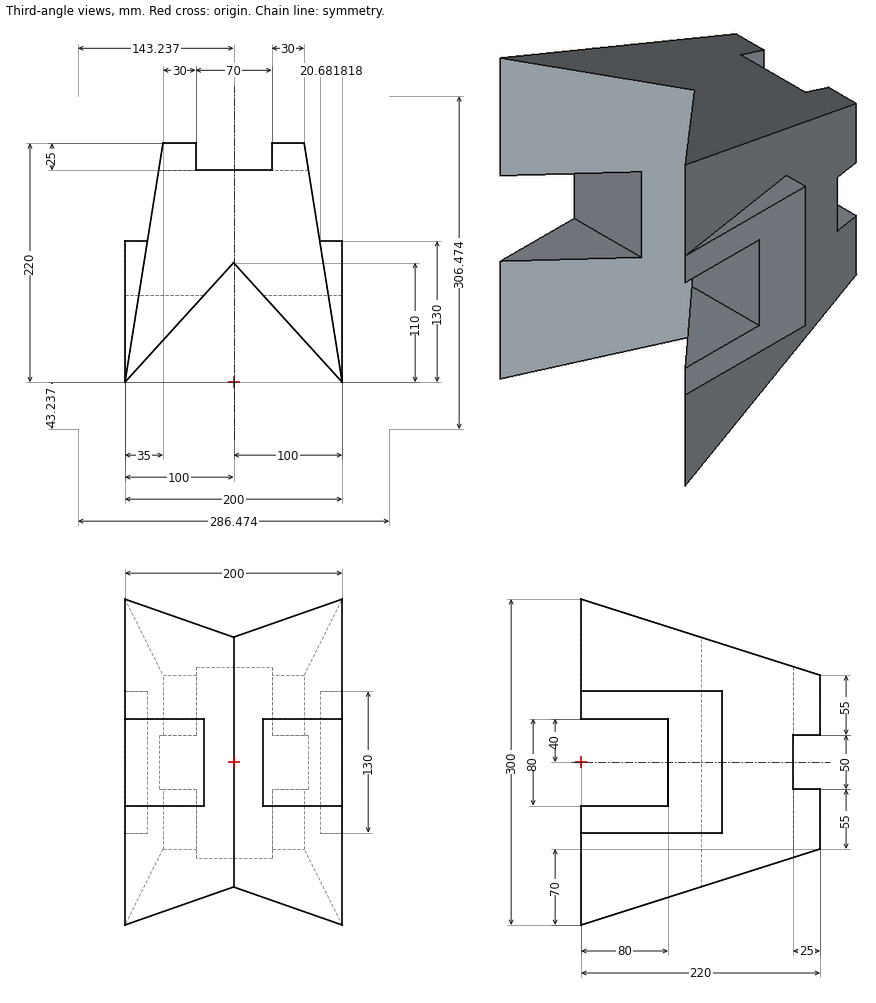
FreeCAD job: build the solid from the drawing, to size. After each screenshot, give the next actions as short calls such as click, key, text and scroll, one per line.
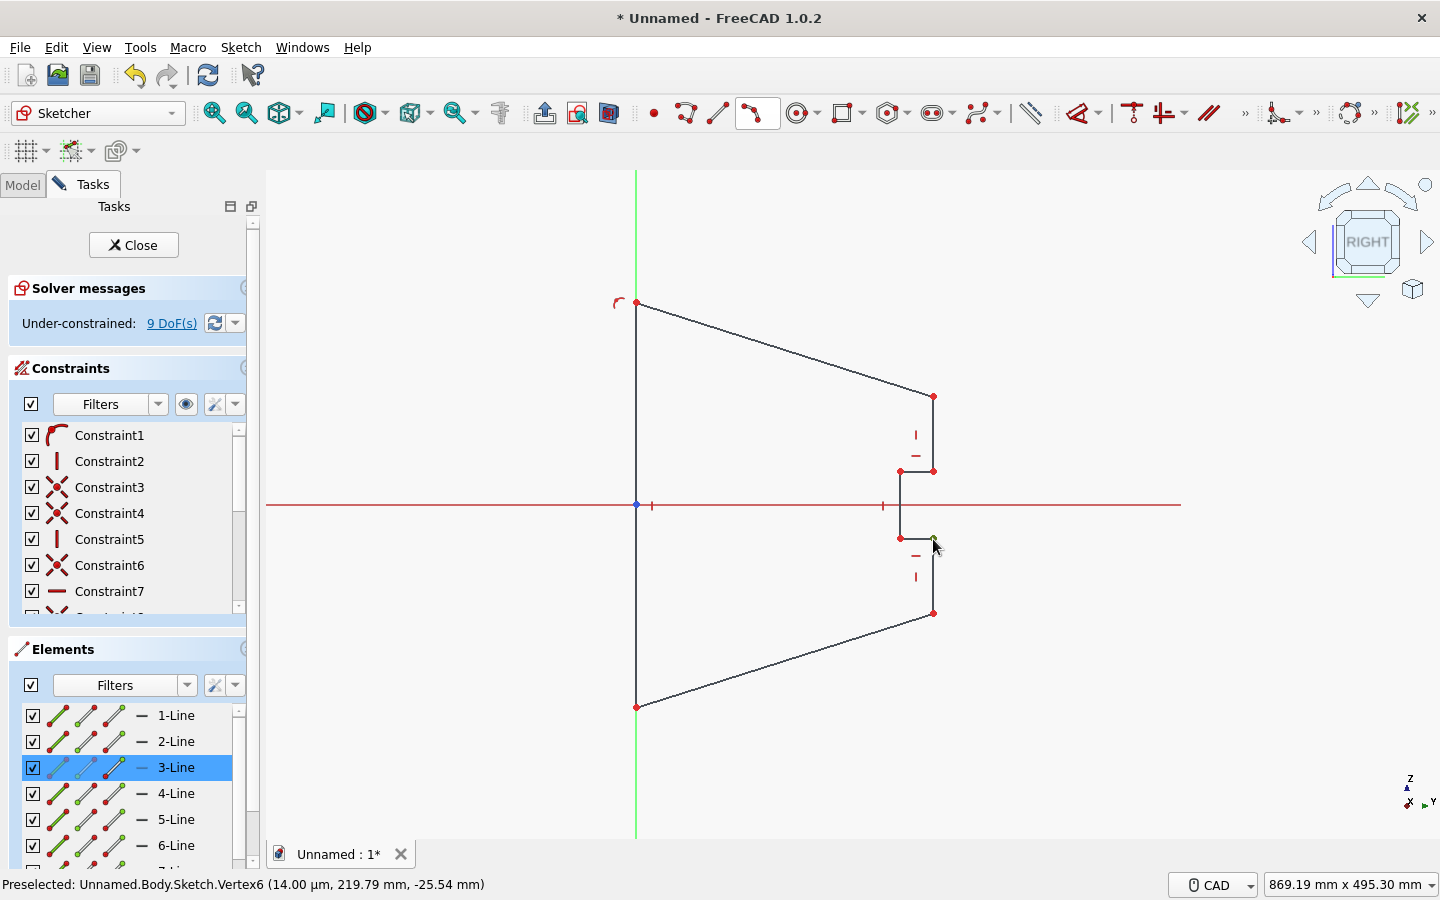
click(933, 472)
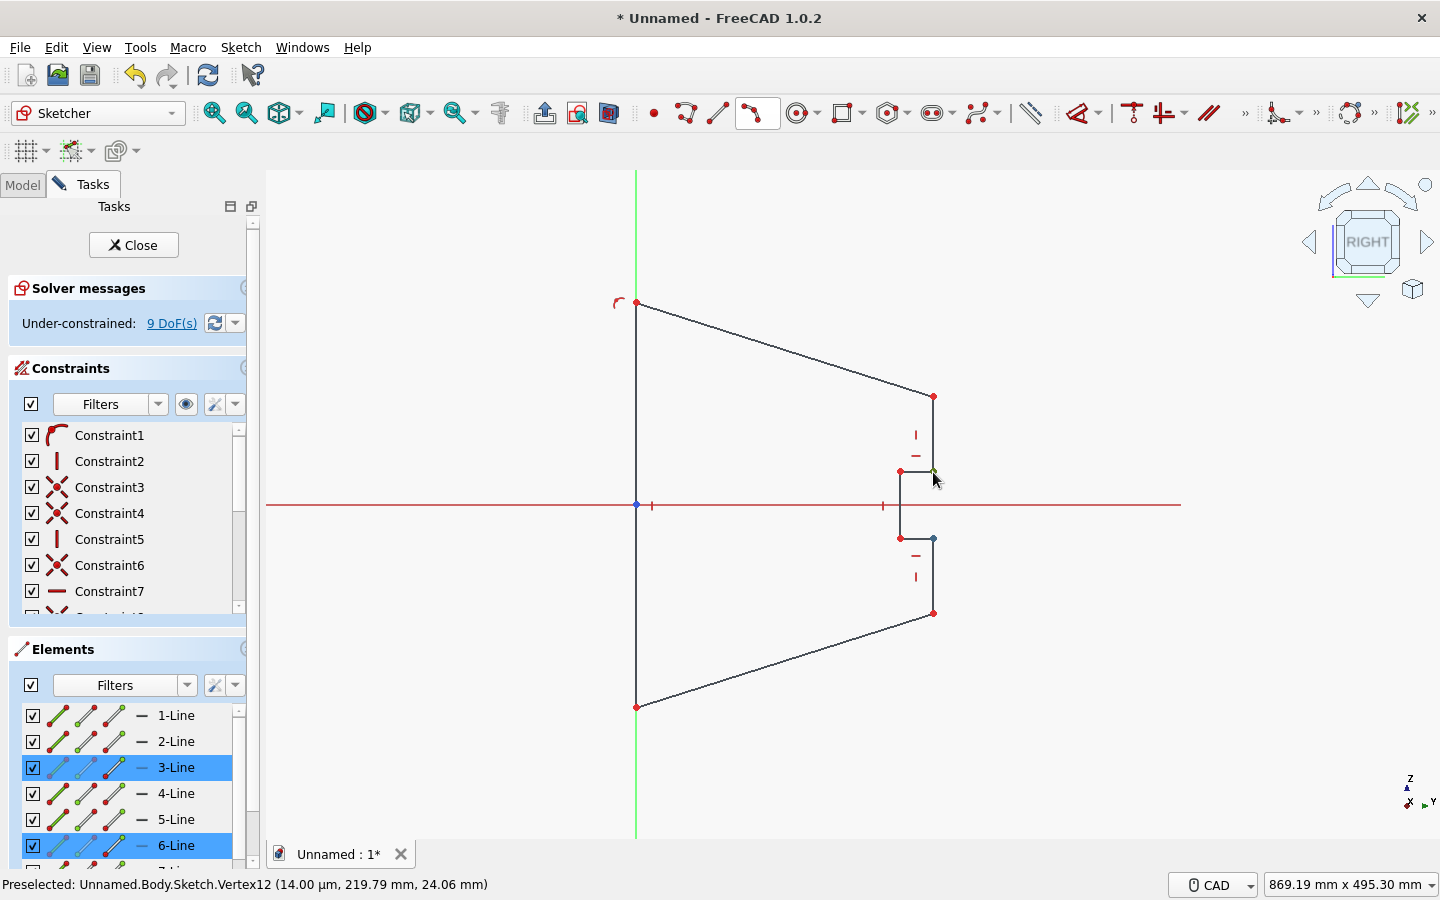
click(364, 504)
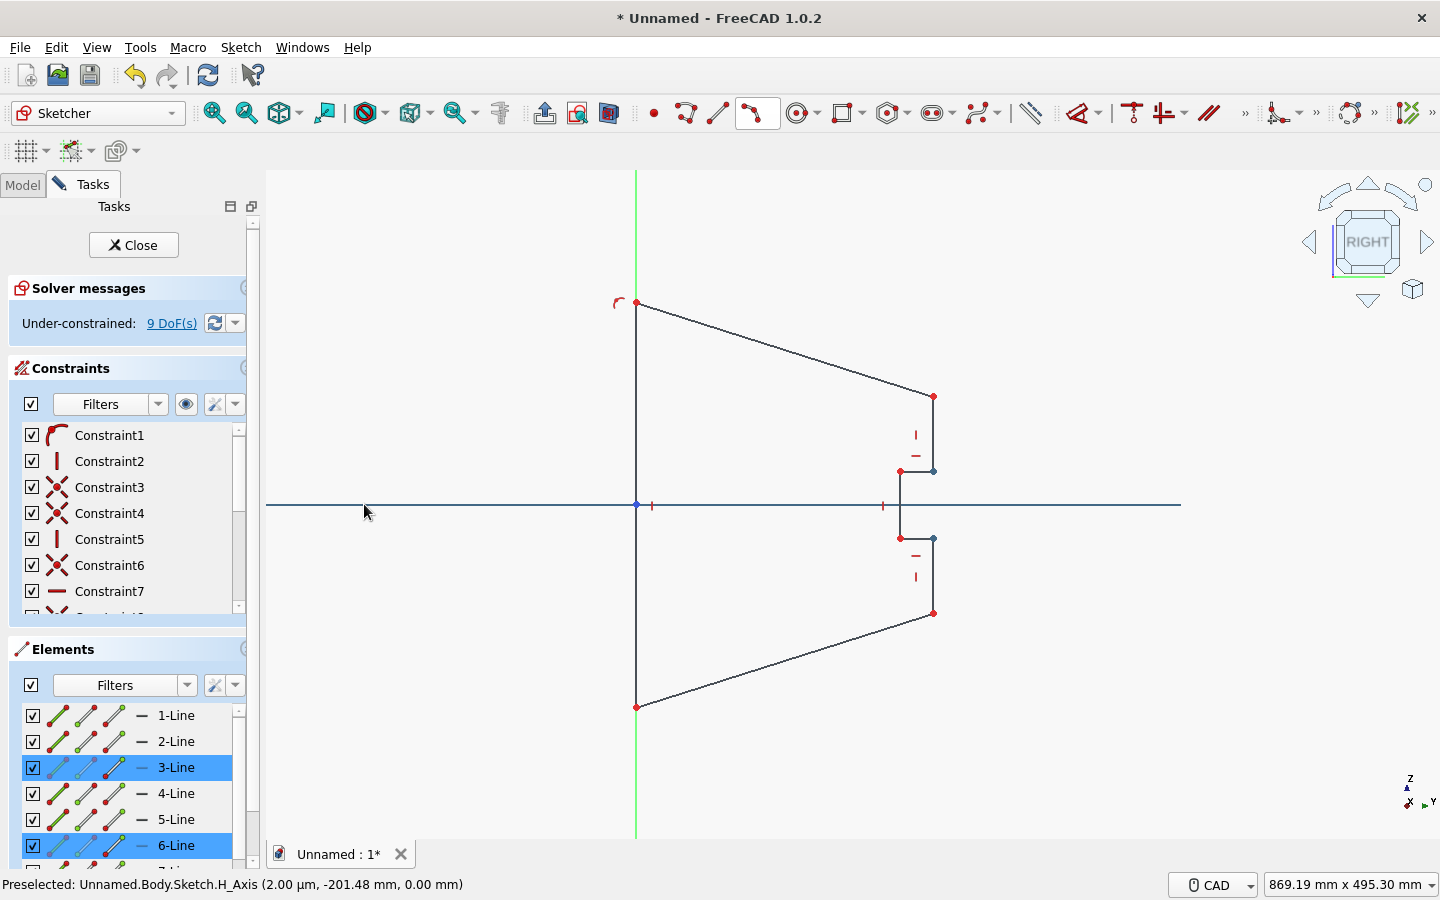
key(s)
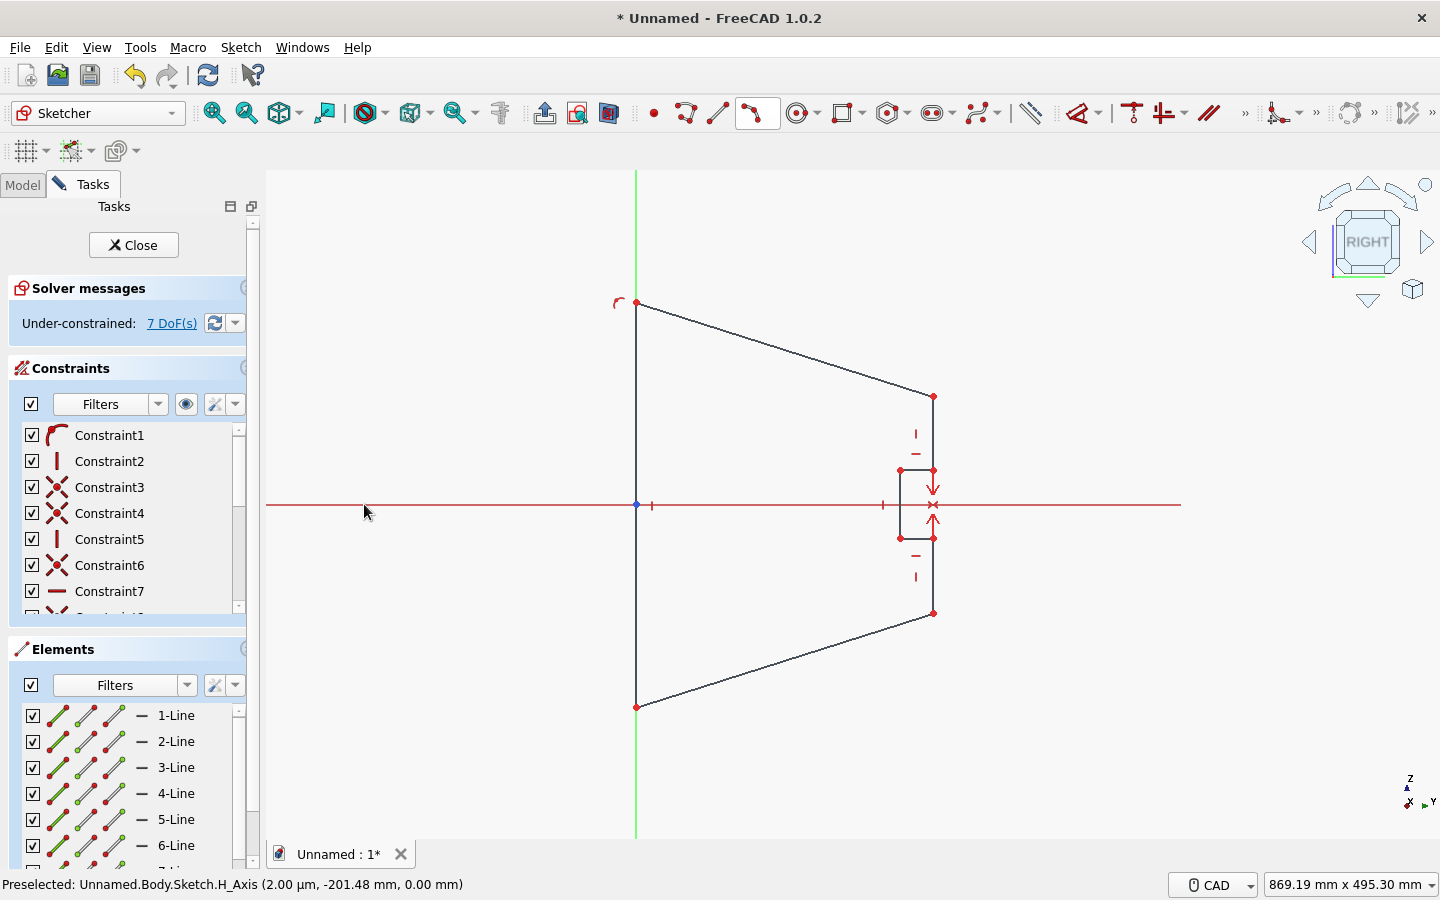
click(933, 591)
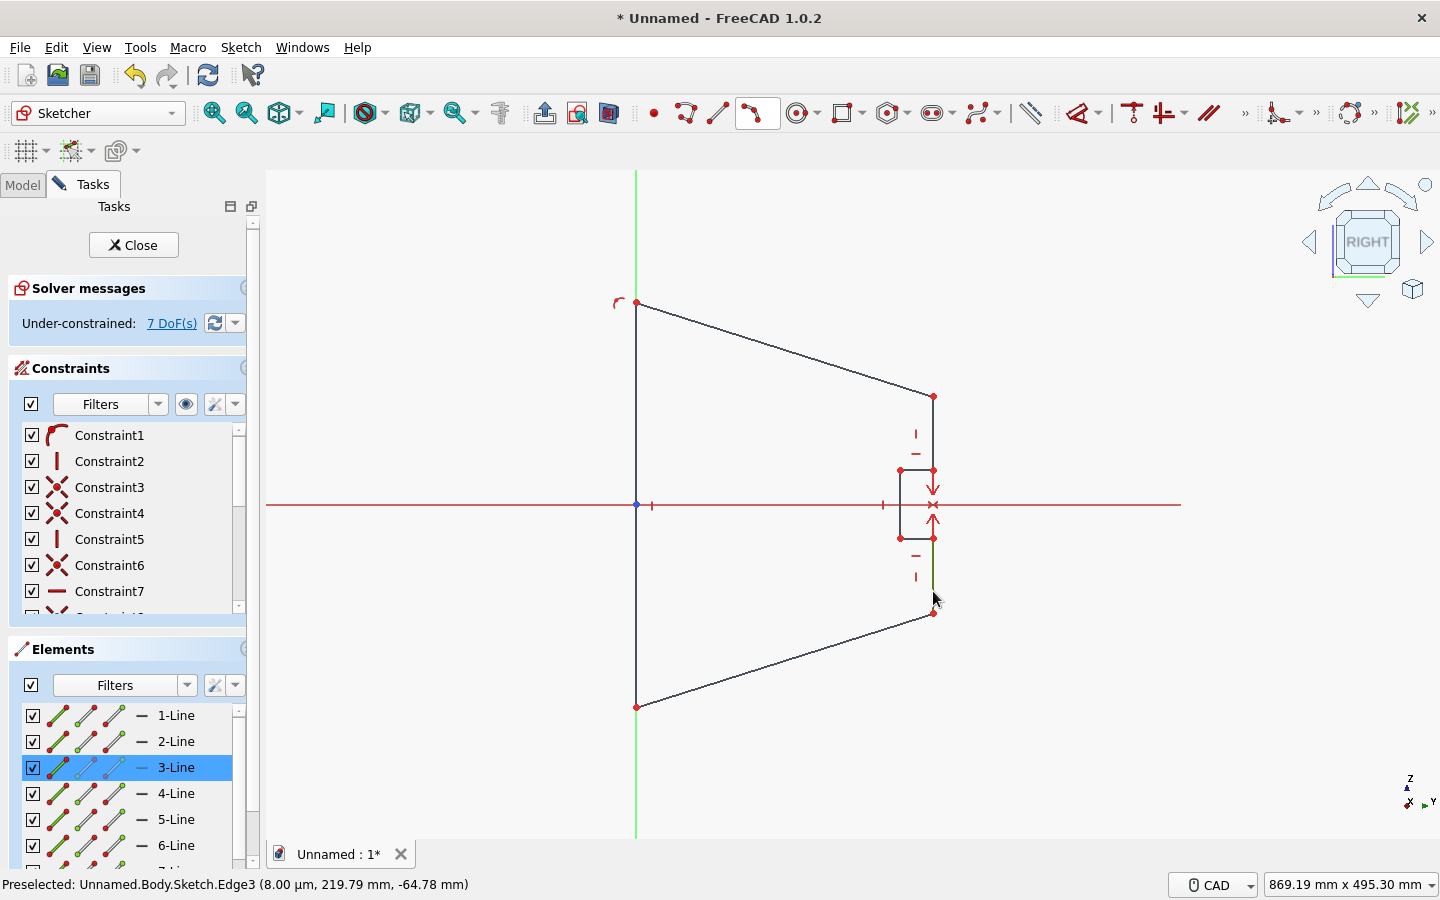
click(1100, 114)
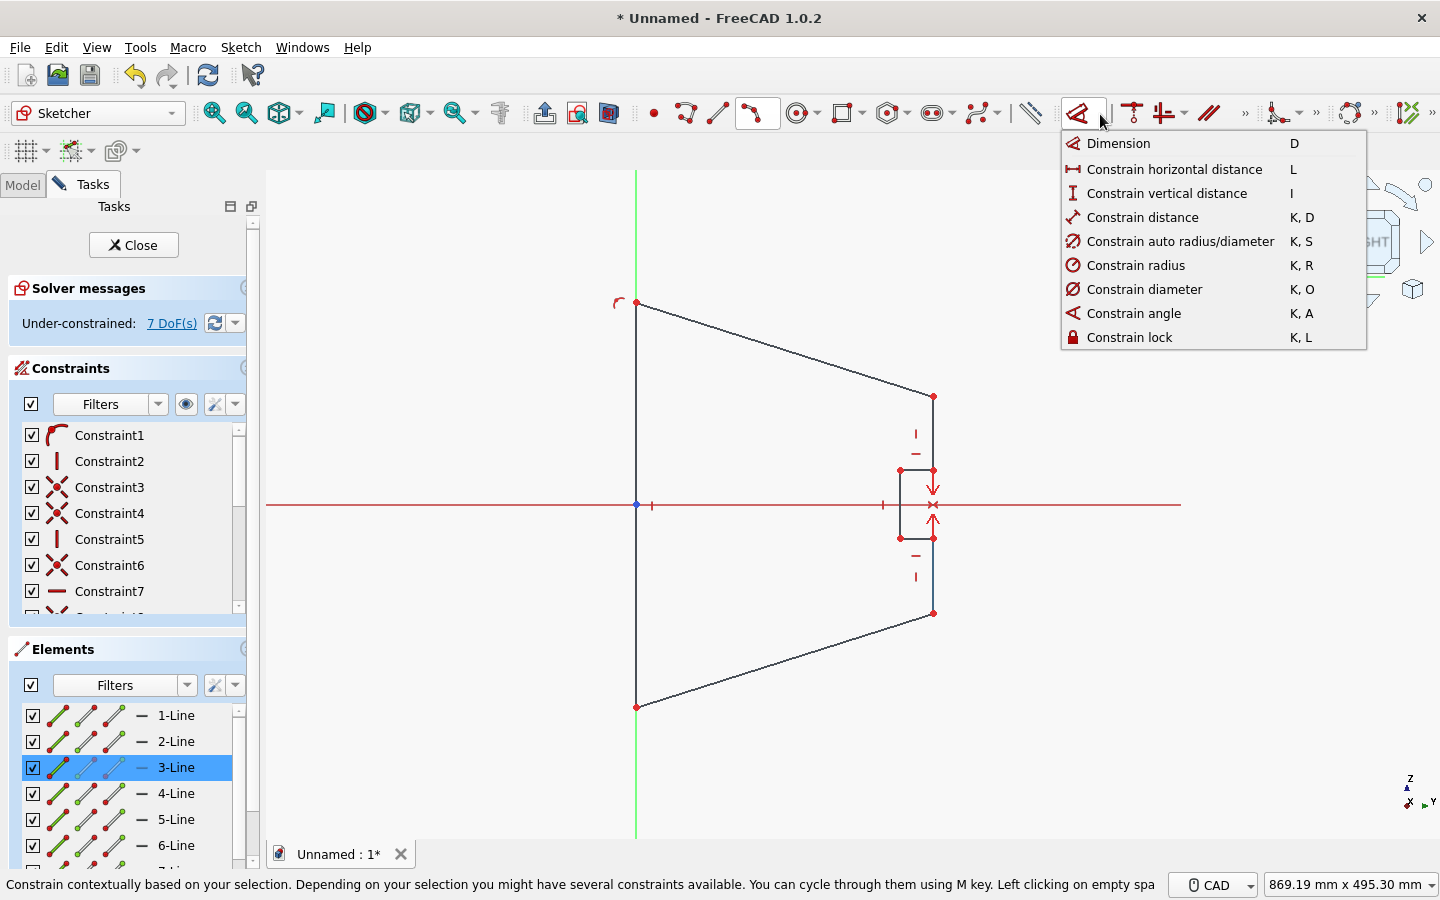
click(1214, 193)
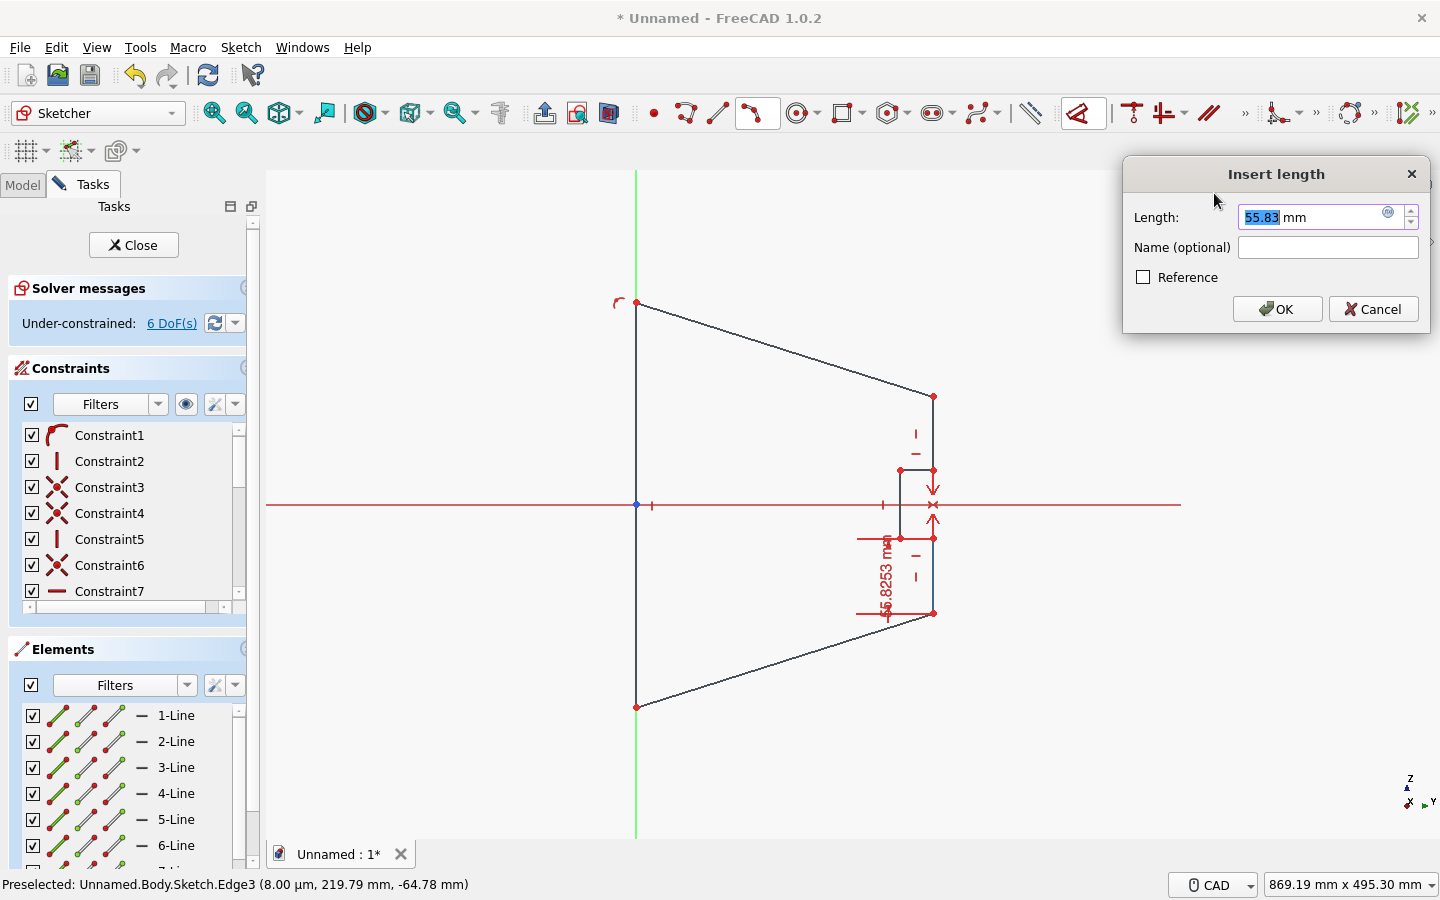
text(55)
key(Return)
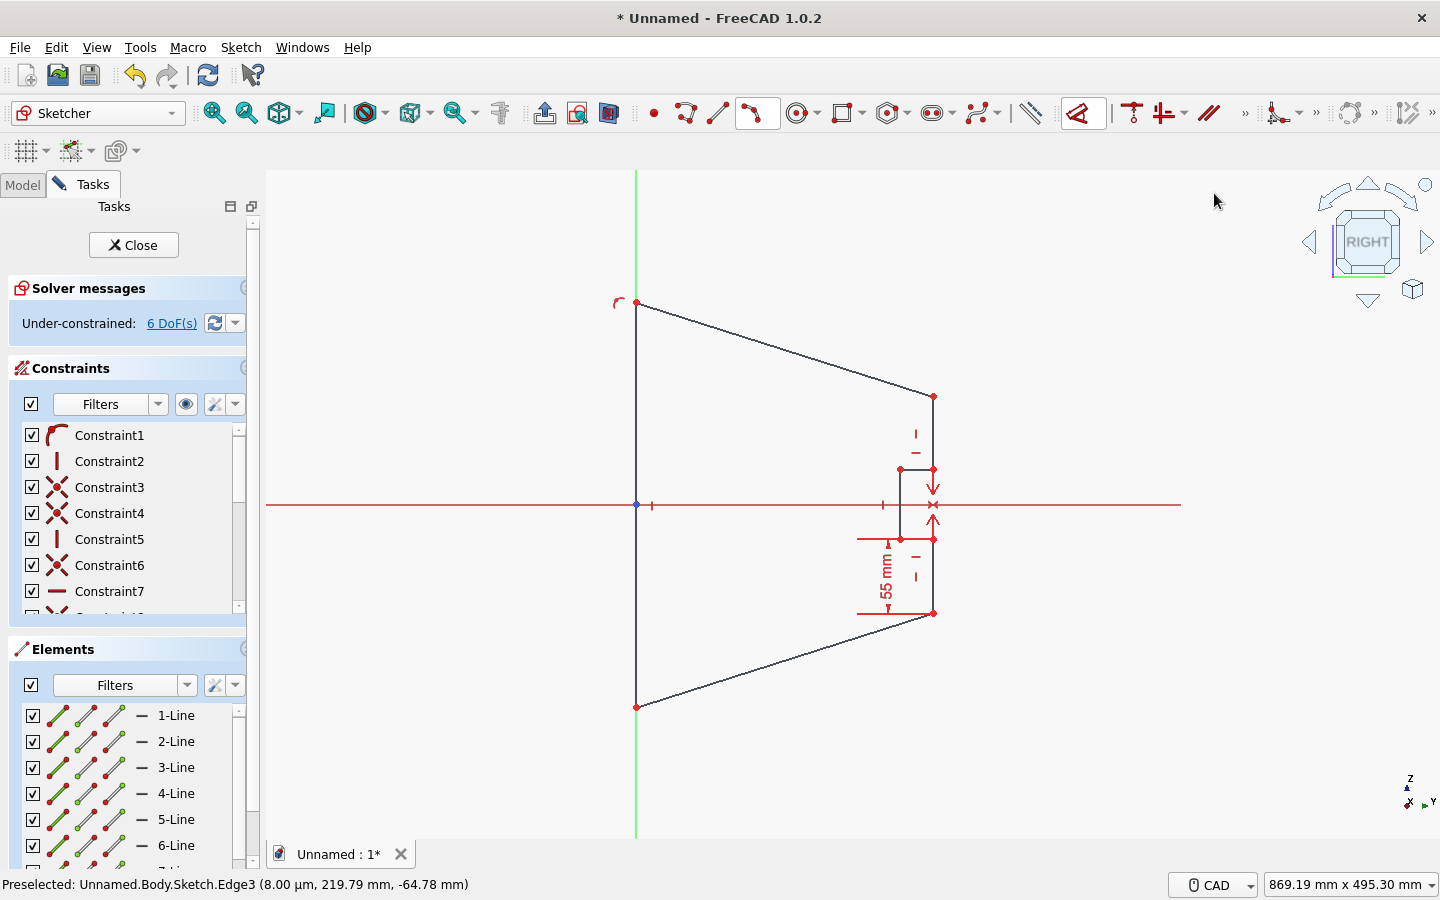
scroll(923, 539, up, 2)